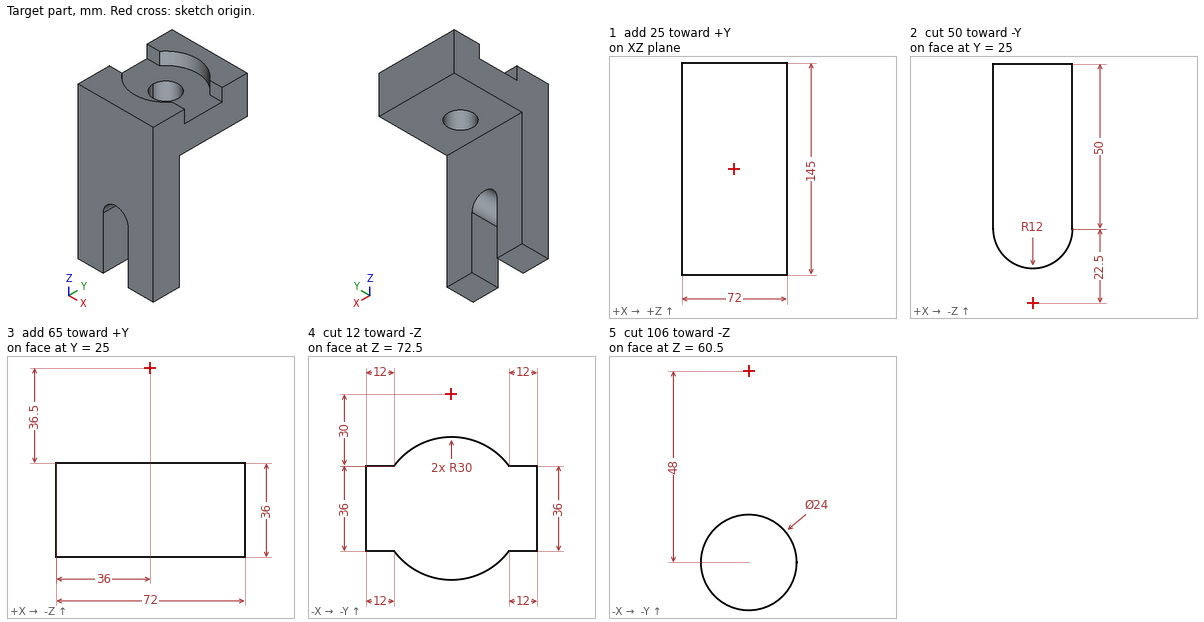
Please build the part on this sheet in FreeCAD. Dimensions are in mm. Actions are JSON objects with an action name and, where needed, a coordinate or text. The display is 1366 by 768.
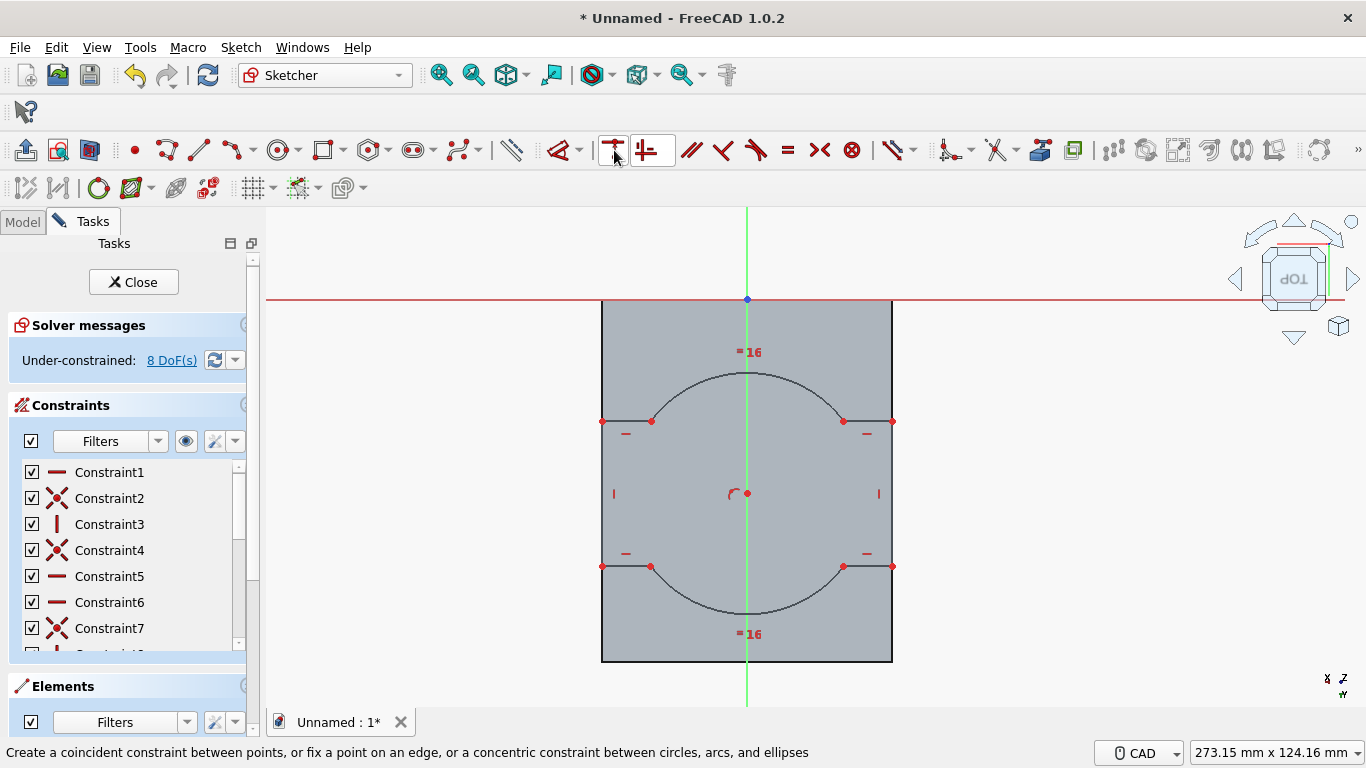
{"action": "left_click", "coordinate": [558, 150]}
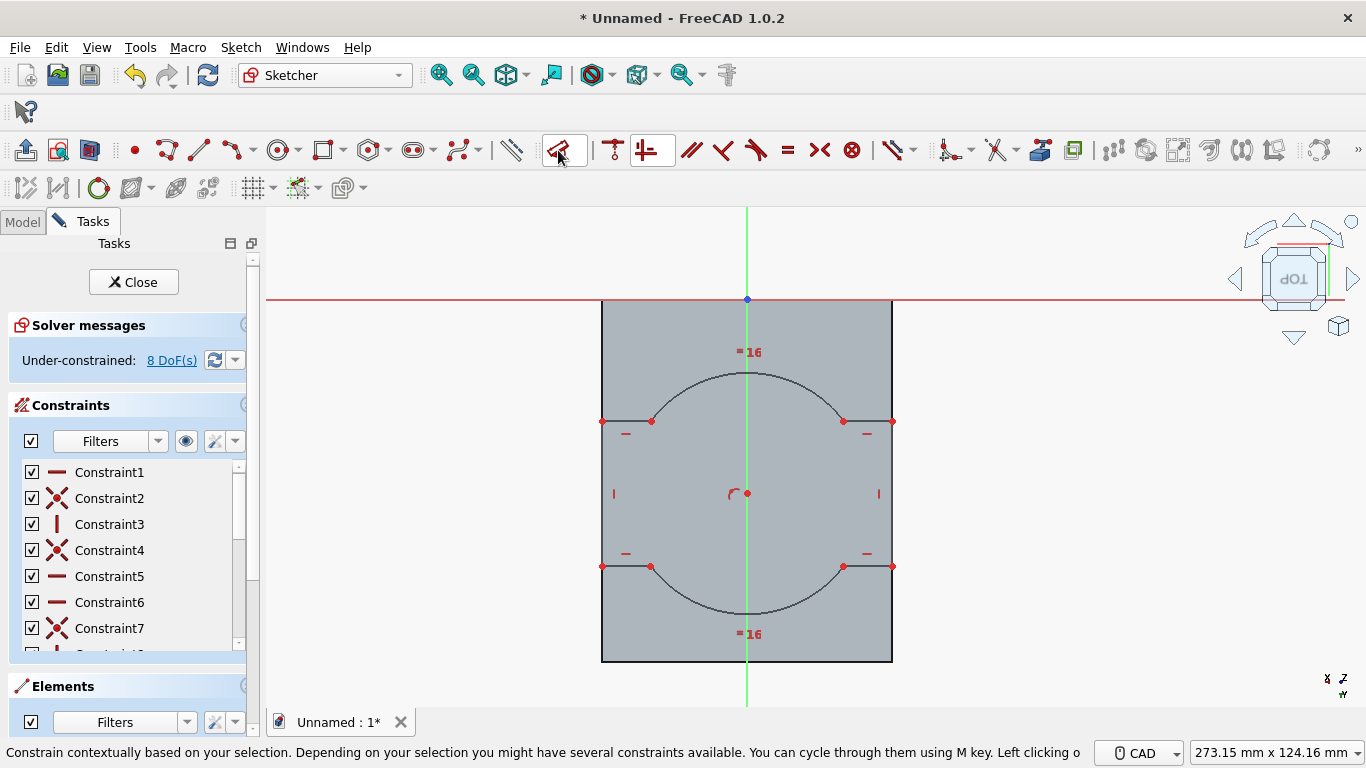
{"action": "left_click", "coordinate": [704, 606]}
{"action": "left_click", "coordinate": [692, 636]}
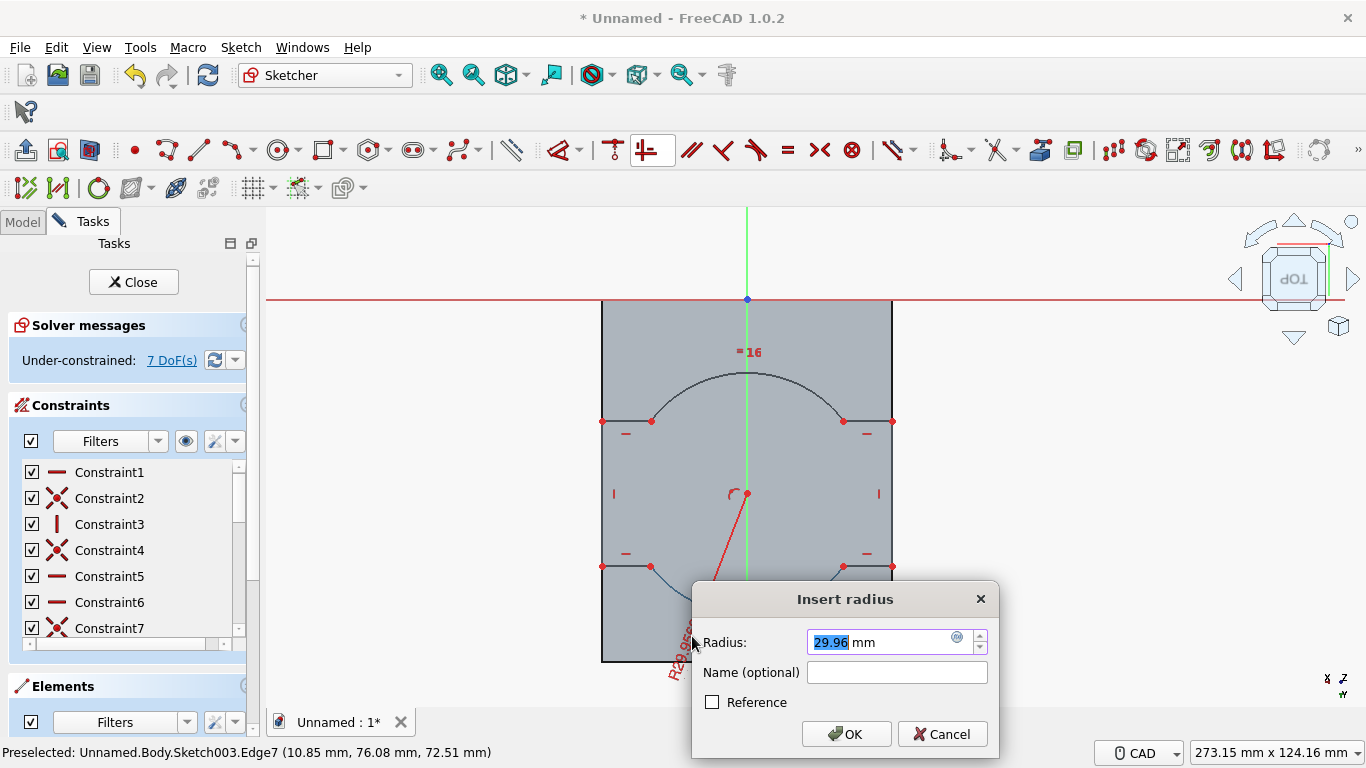
{"action": "type", "text": "30"}
{"action": "key", "text": "Return"}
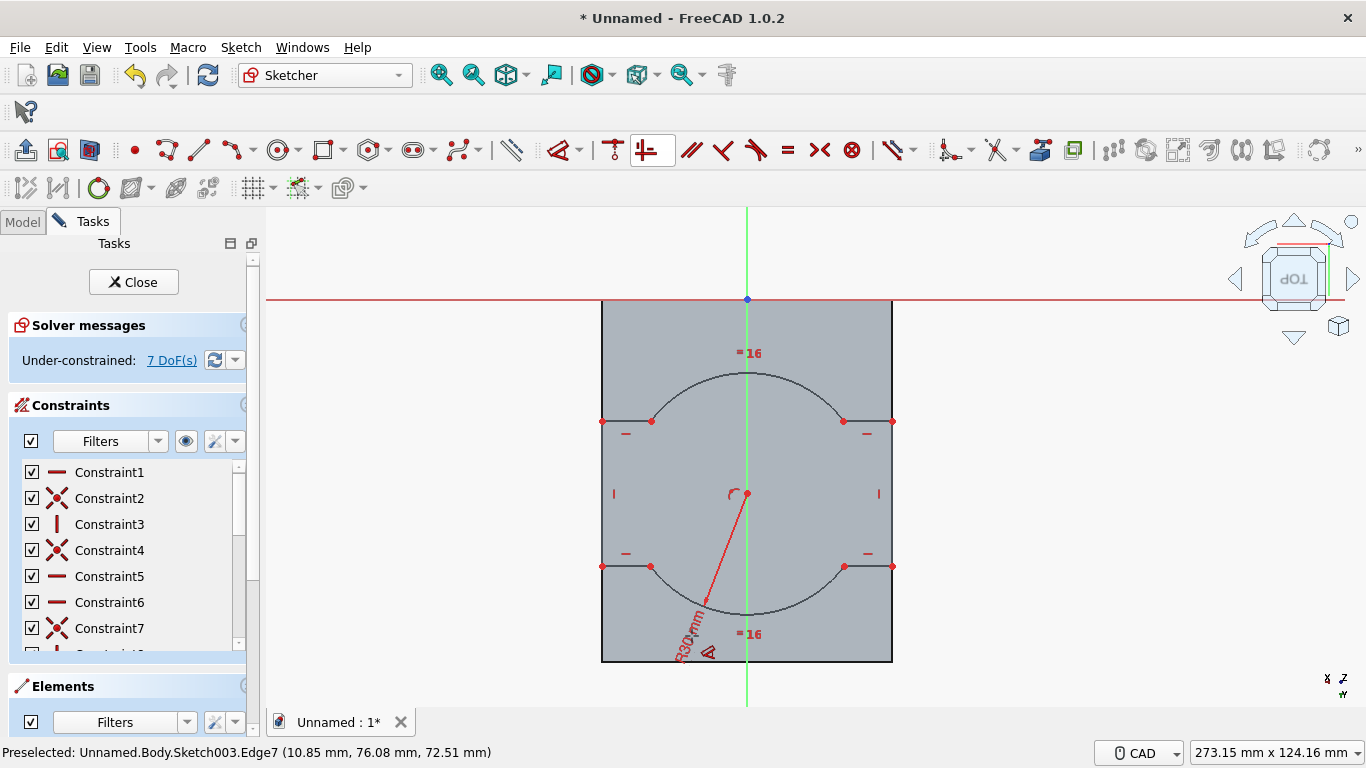
{"action": "left_click", "coordinate": [636, 421]}
{"action": "left_click", "coordinate": [627, 387]}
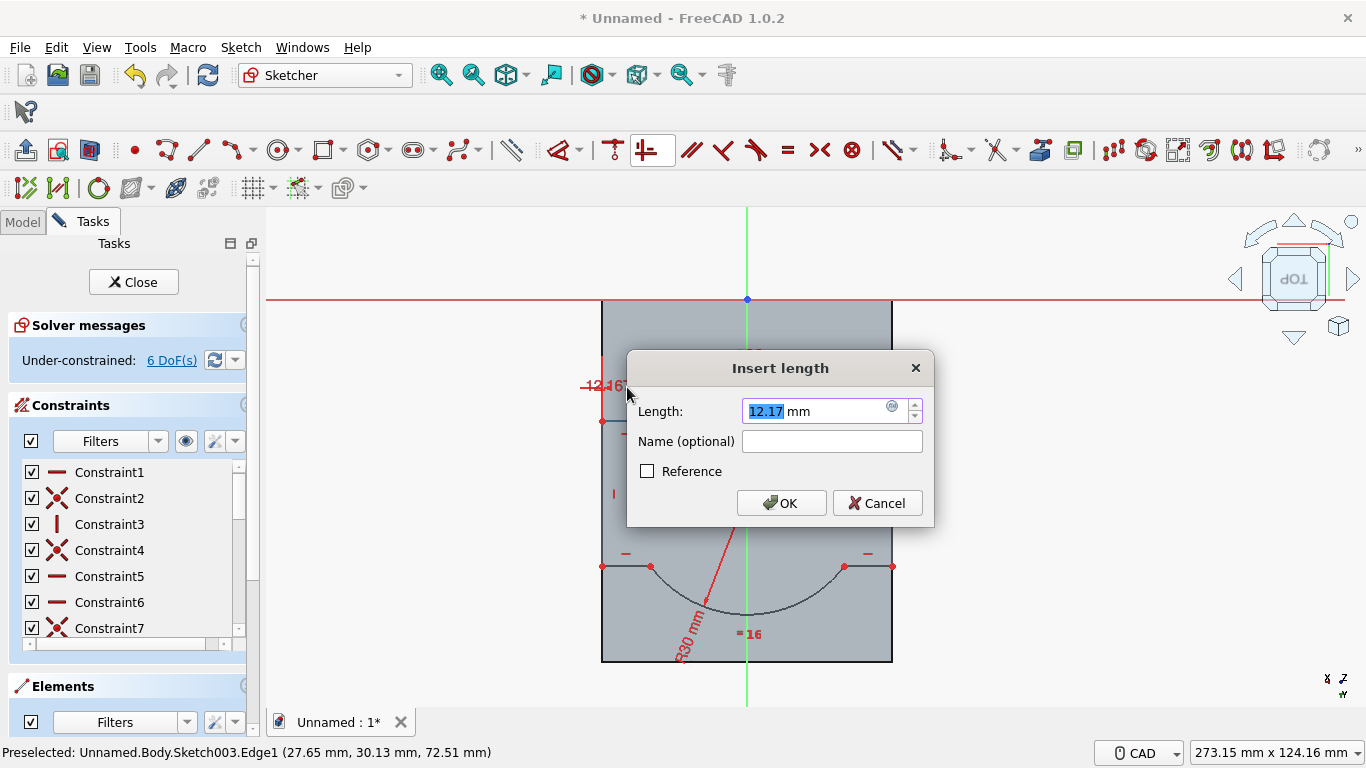
{"action": "type", "text": "12"}
{"action": "key", "text": "Return"}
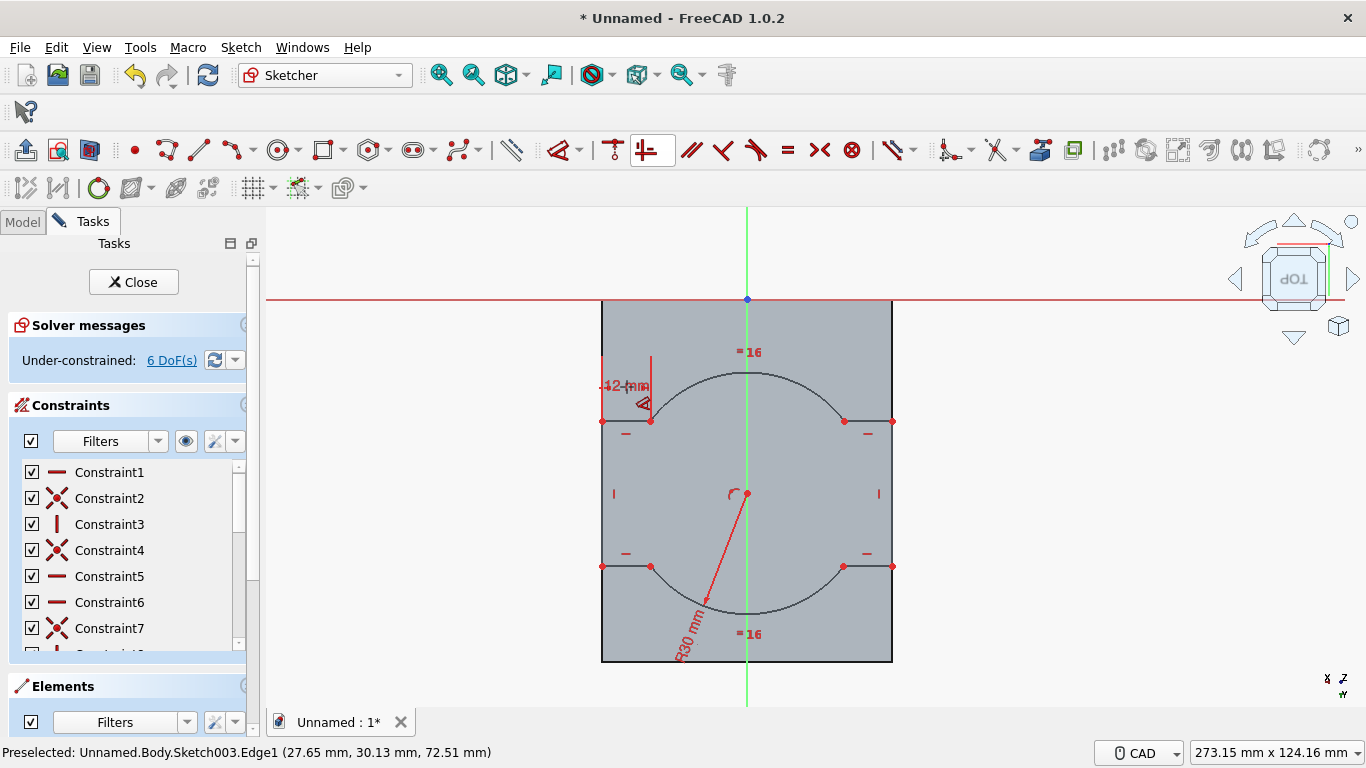
{"action": "left_click", "coordinate": [602, 465]}
{"action": "left_click", "coordinate": [568, 494]}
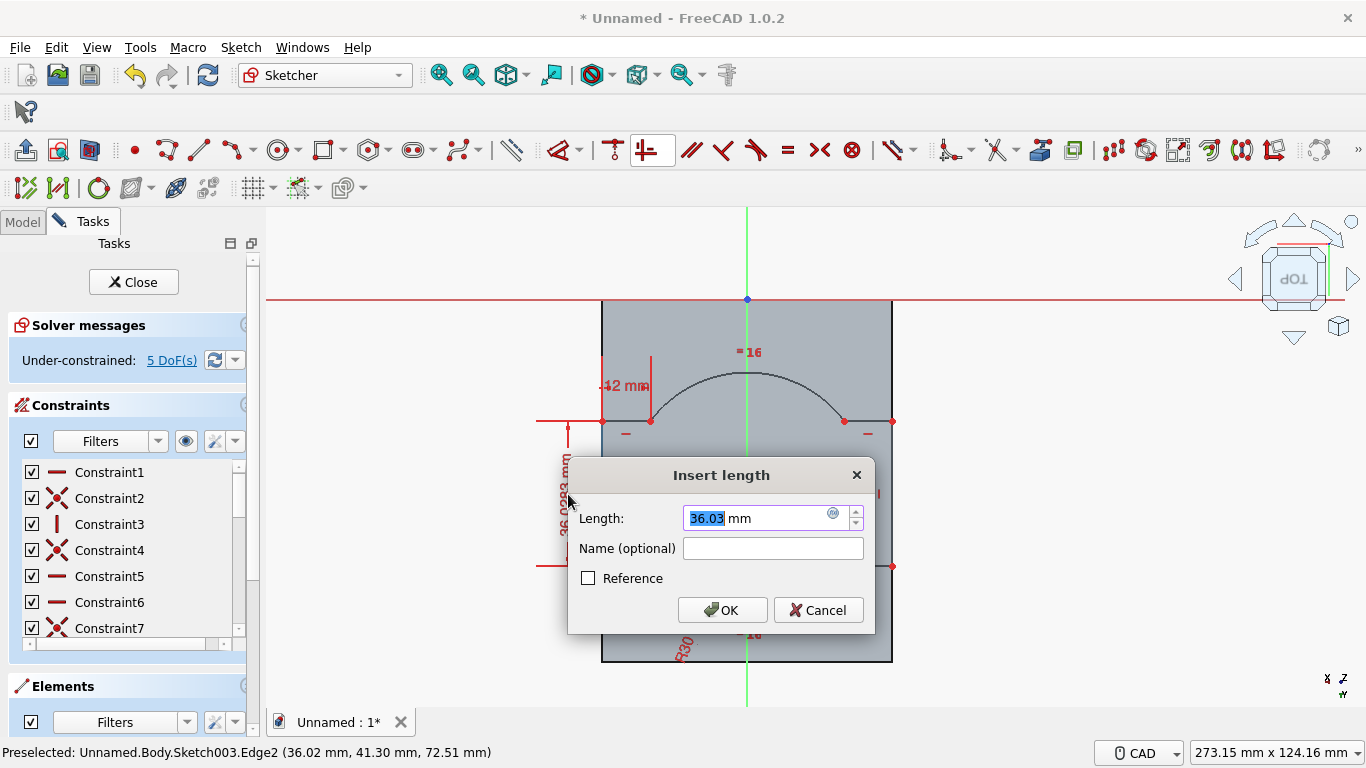
{"action": "type", "text": "36"}
{"action": "key", "text": "Return"}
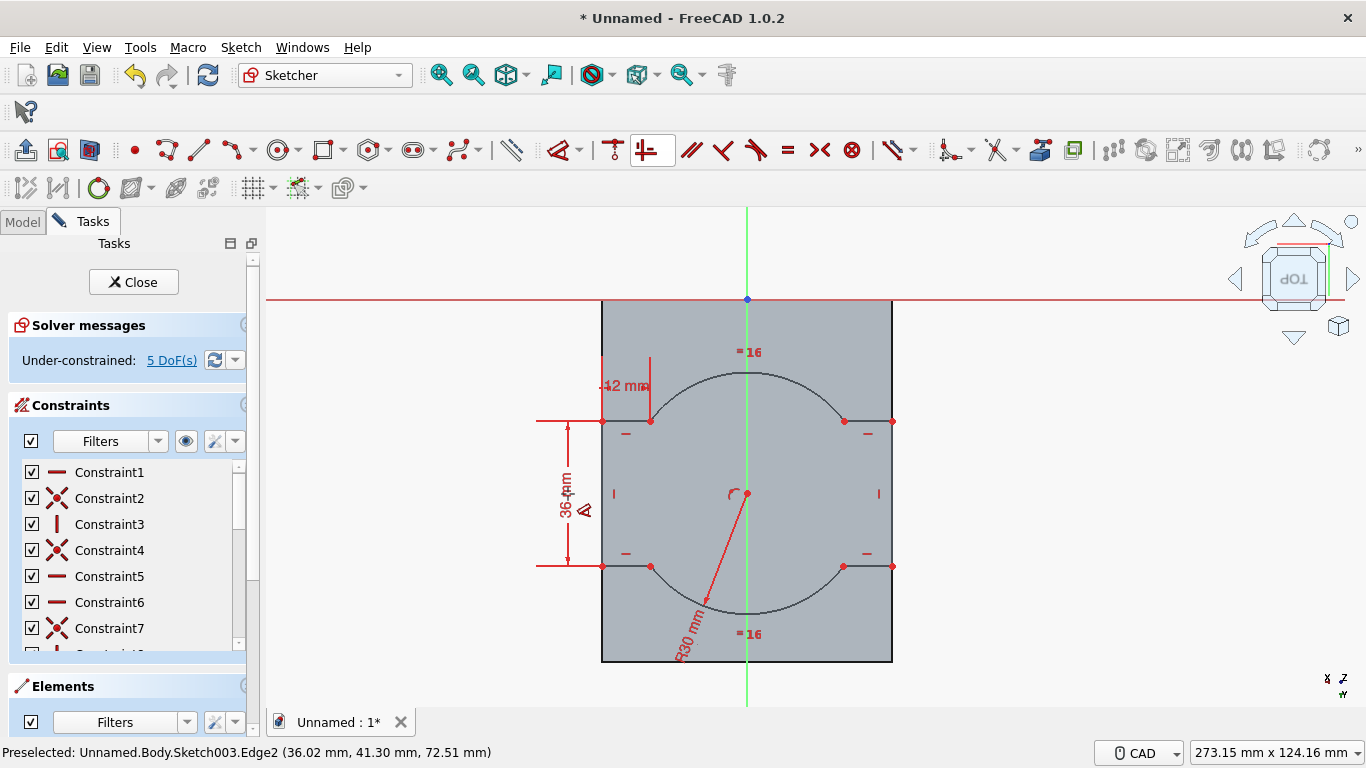
{"action": "left_click", "coordinate": [617, 566]}
{"action": "left_click", "coordinate": [627, 600]}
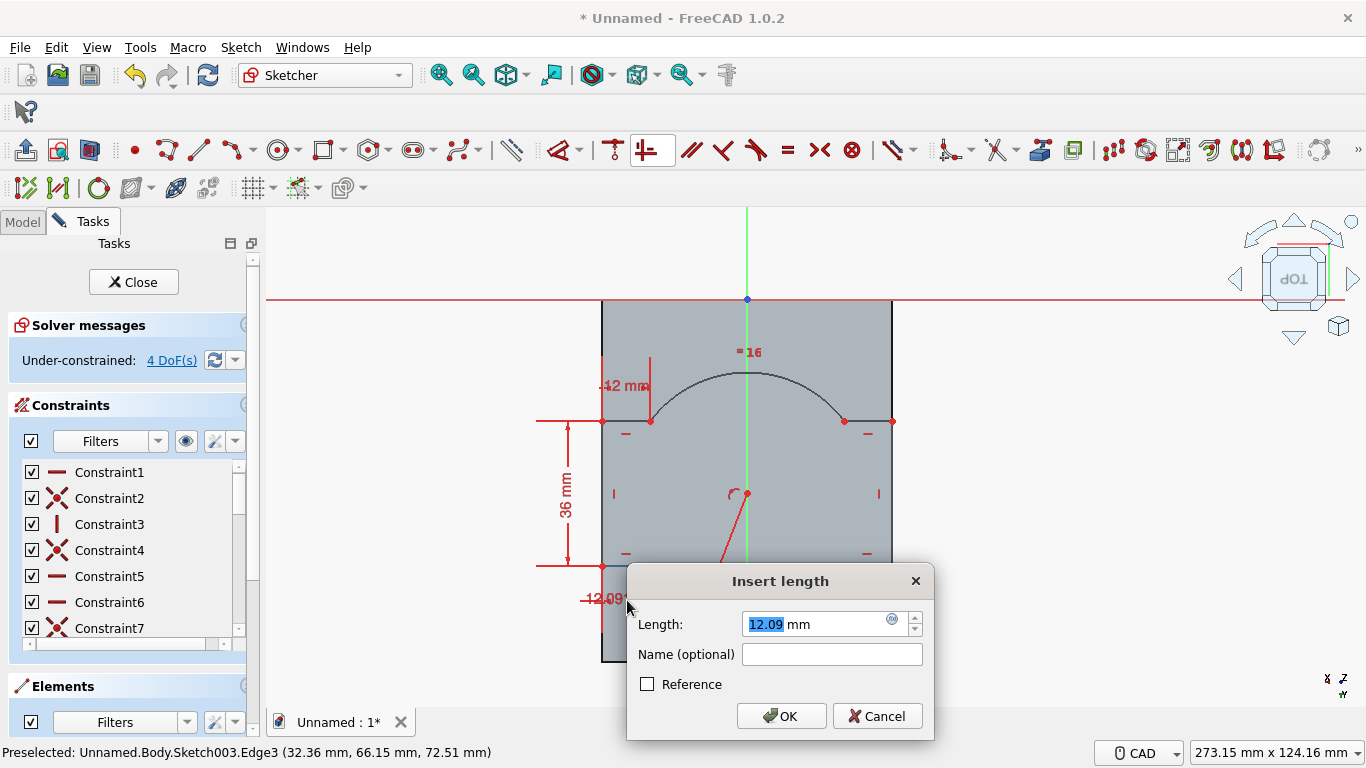
{"action": "type", "text": "12"}
{"action": "key", "text": "Return"}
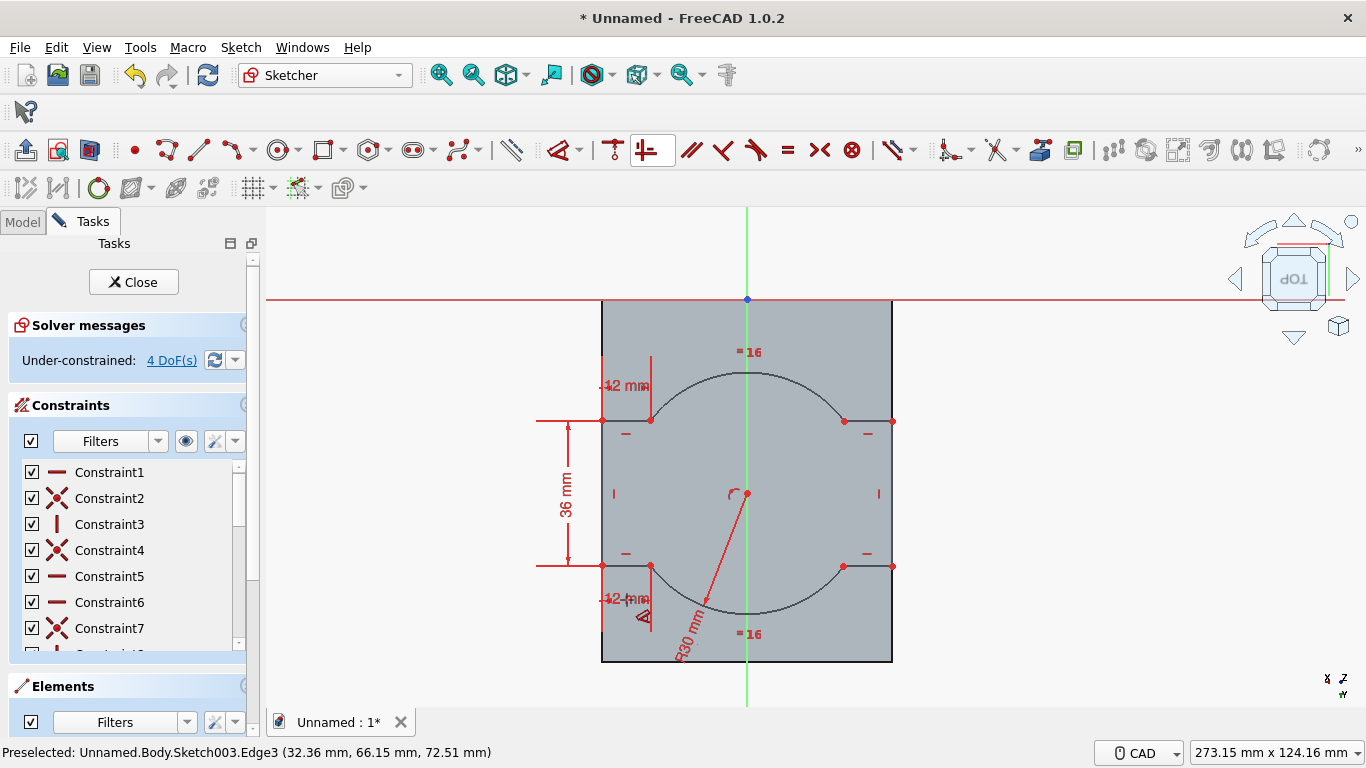
{"action": "left_click", "coordinate": [858, 566]}
{"action": "left_click", "coordinate": [868, 600]}